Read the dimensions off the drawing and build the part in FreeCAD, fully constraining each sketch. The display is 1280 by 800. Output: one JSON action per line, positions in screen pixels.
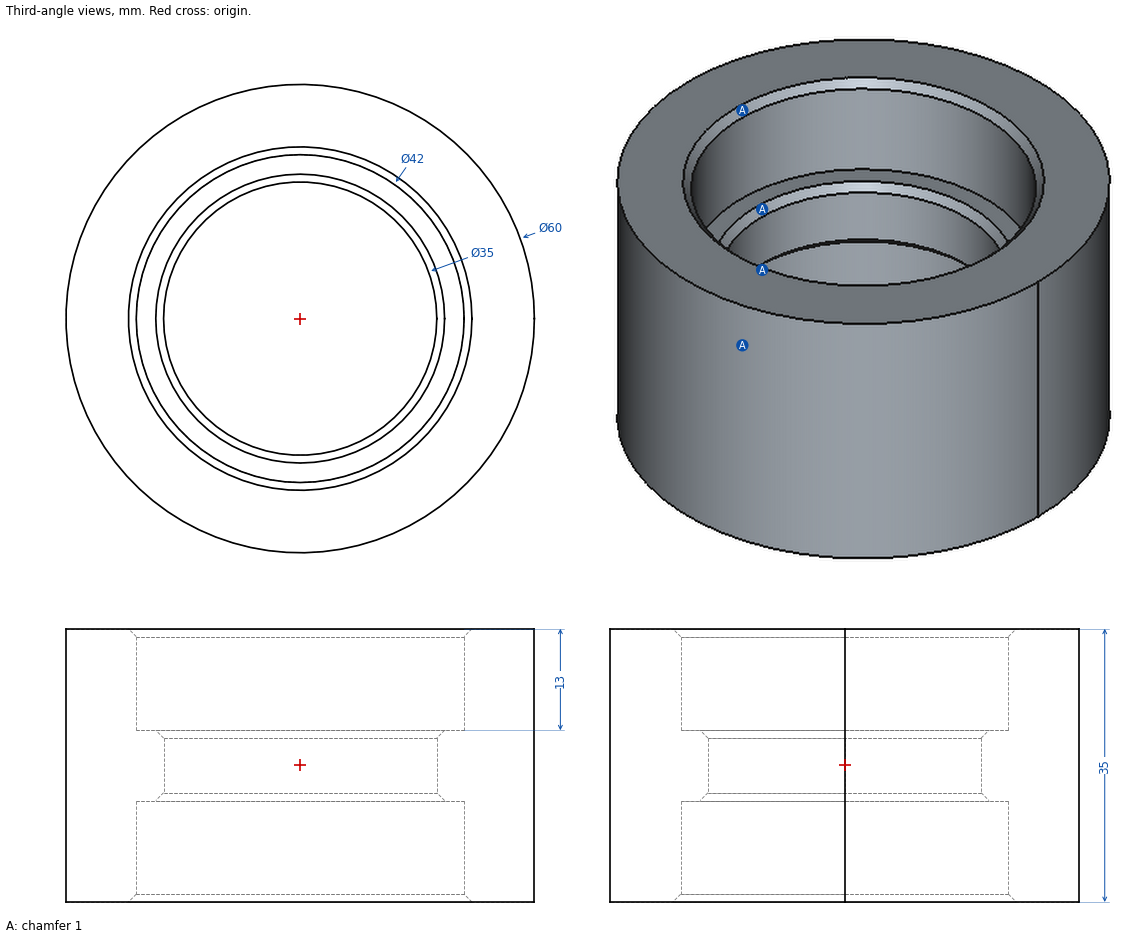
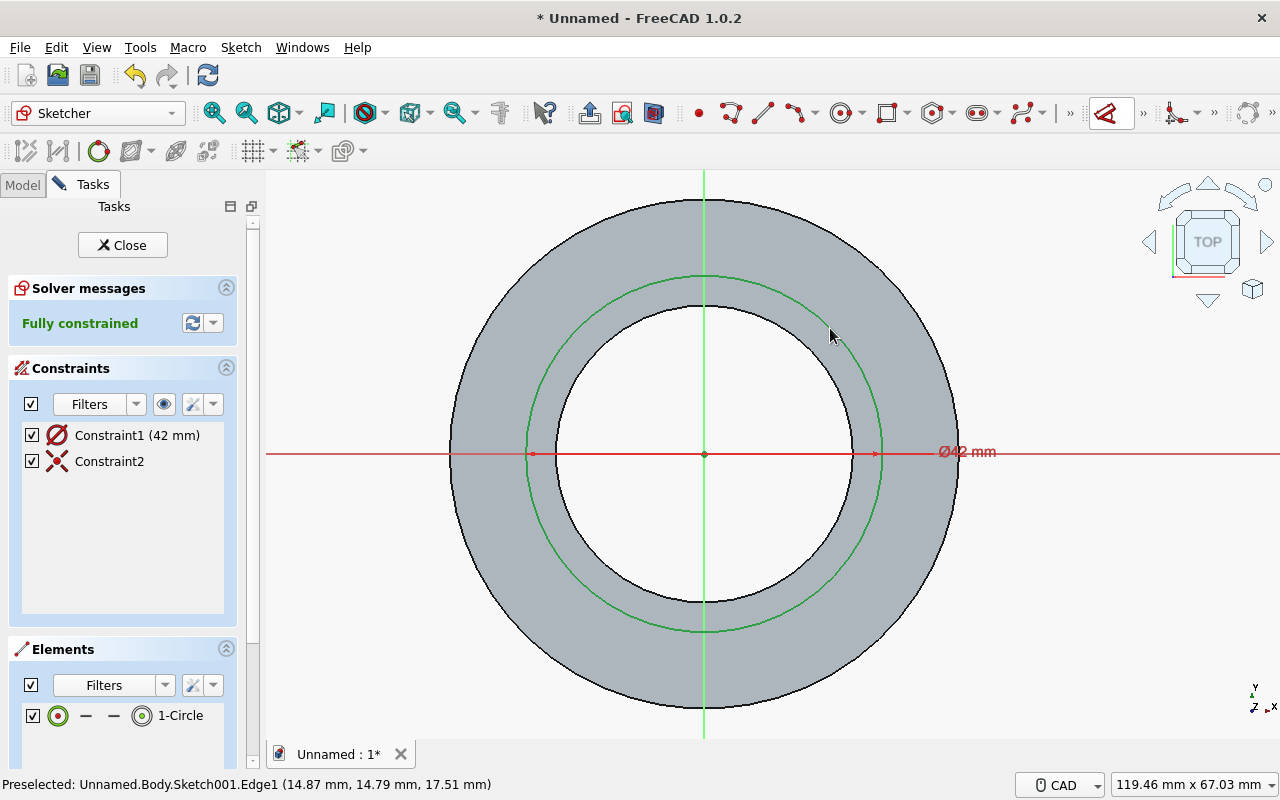
{"action": "left_click", "coordinate": [123, 245]}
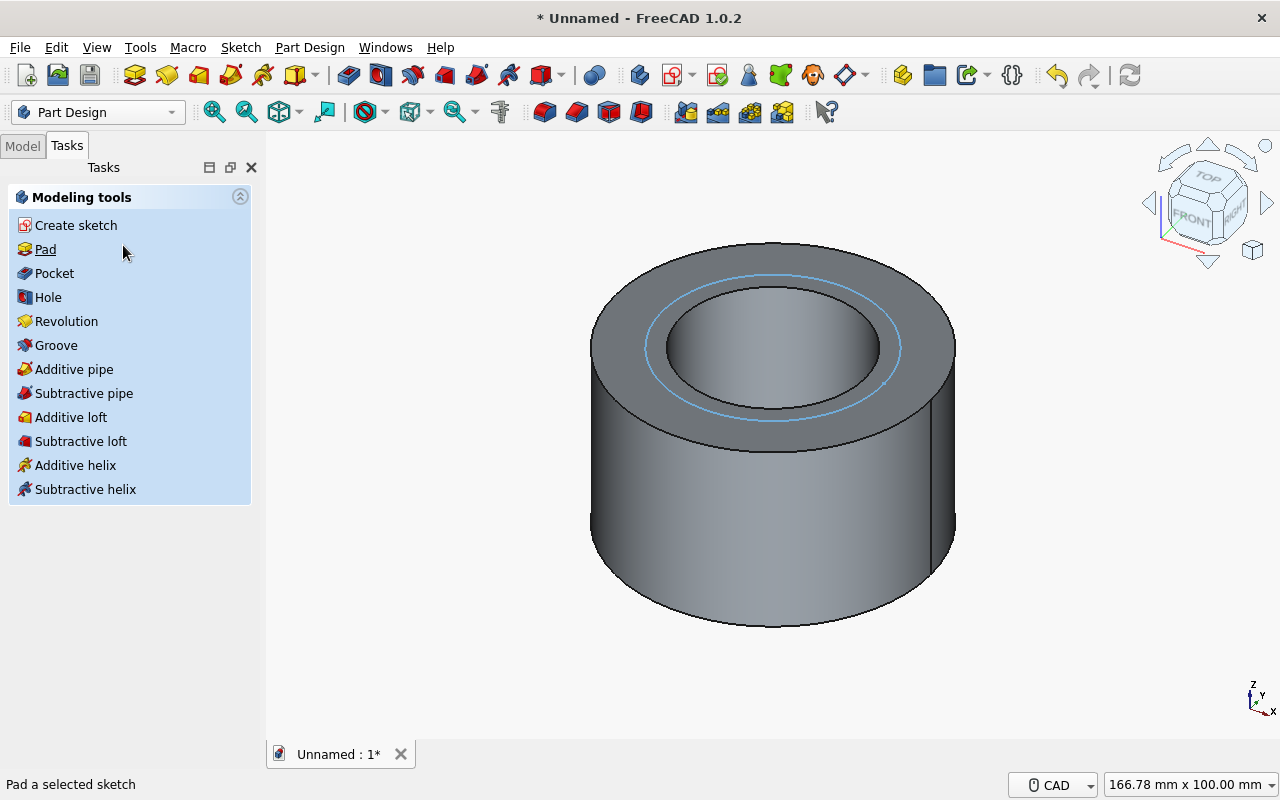
{"action": "left_click", "coordinate": [350, 76]}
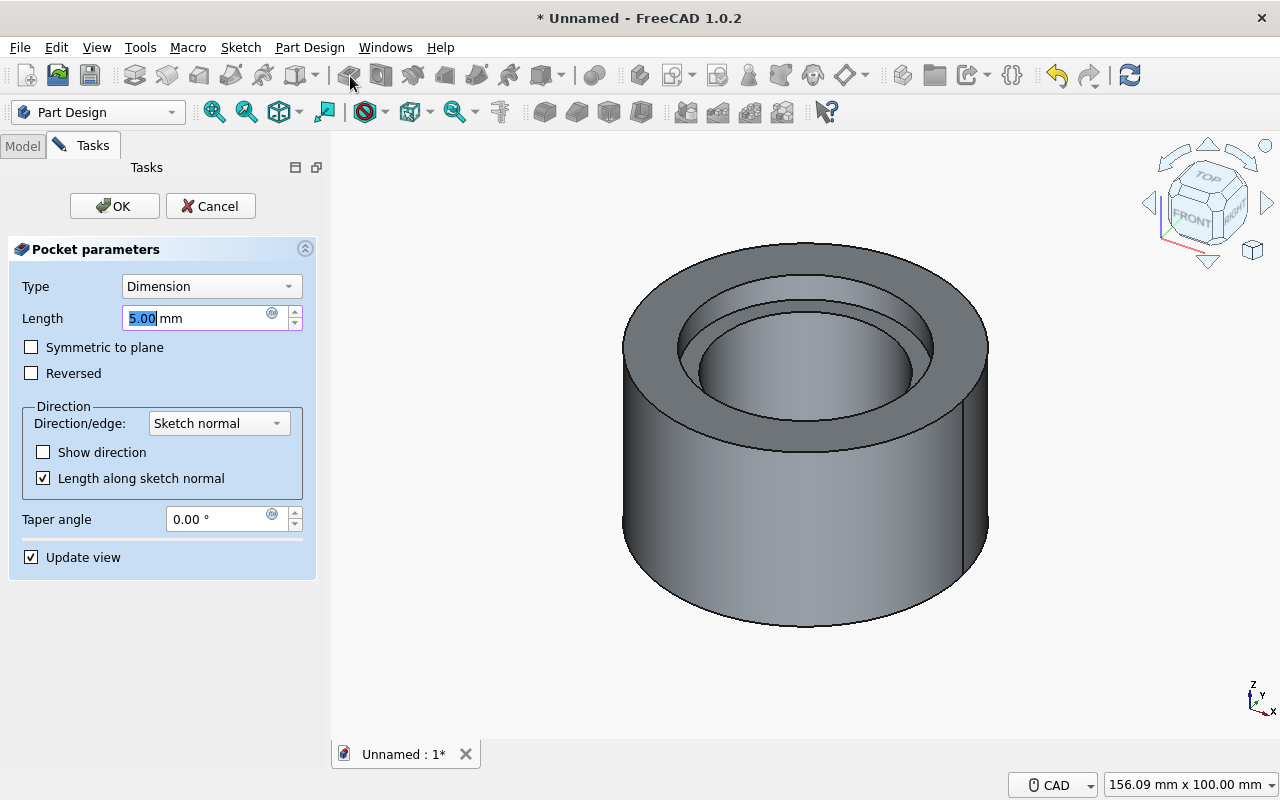
{"action": "type", "text": "13"}
{"action": "key", "text": "Tab"}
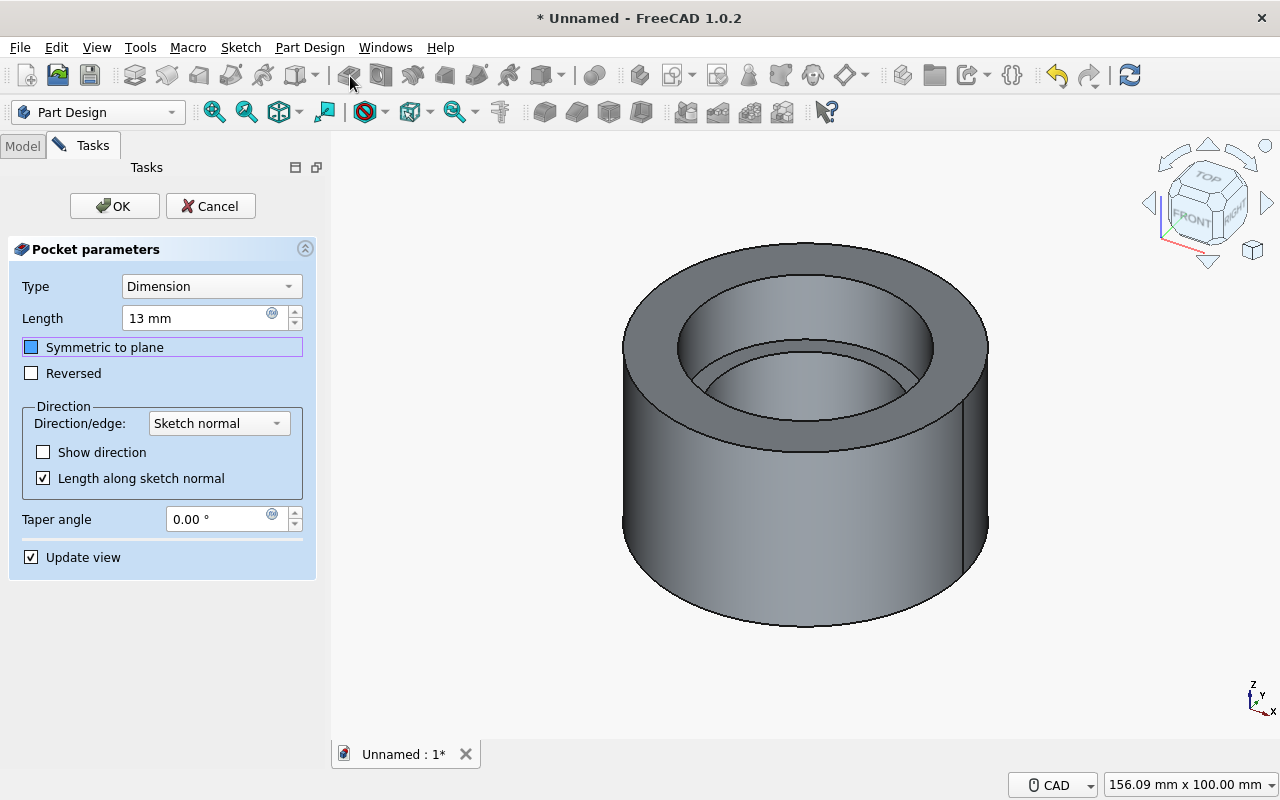
{"action": "left_click", "coordinate": [115, 206]}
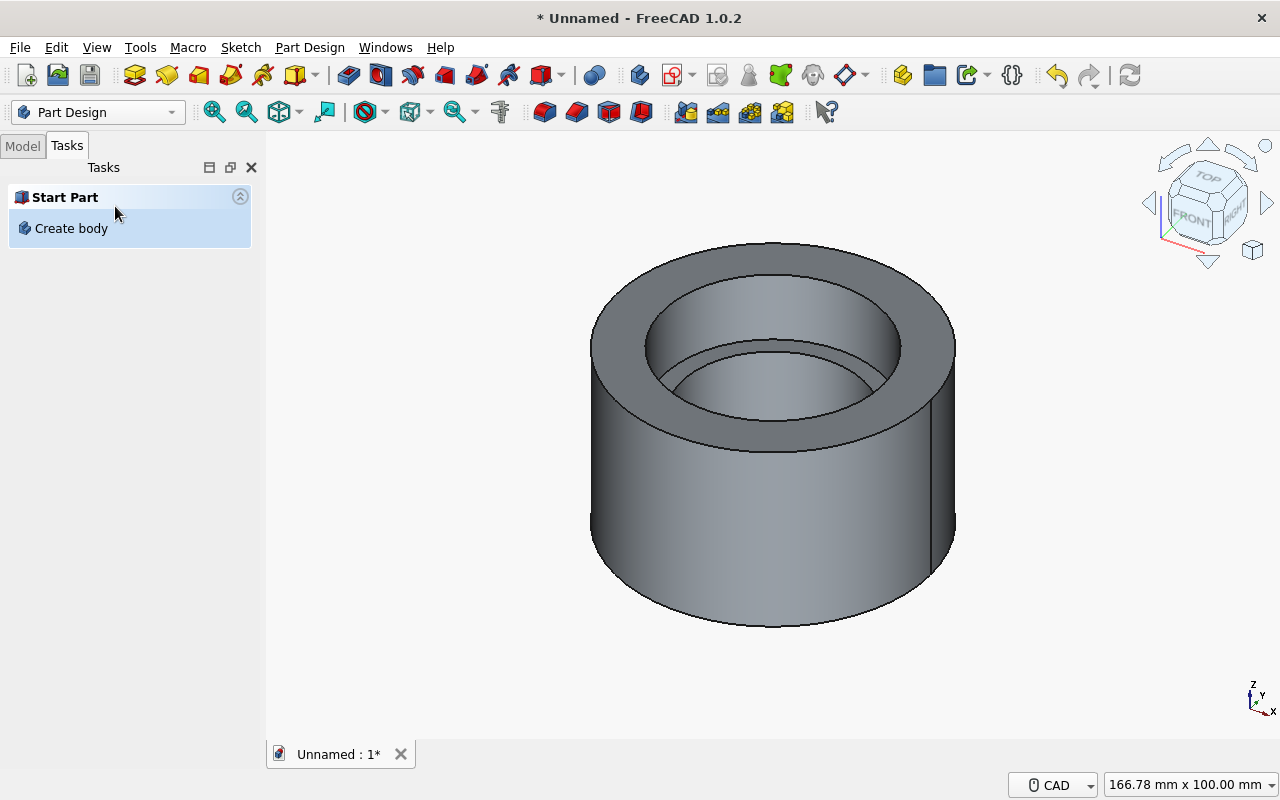
{"action": "left_click", "coordinate": [23, 145]}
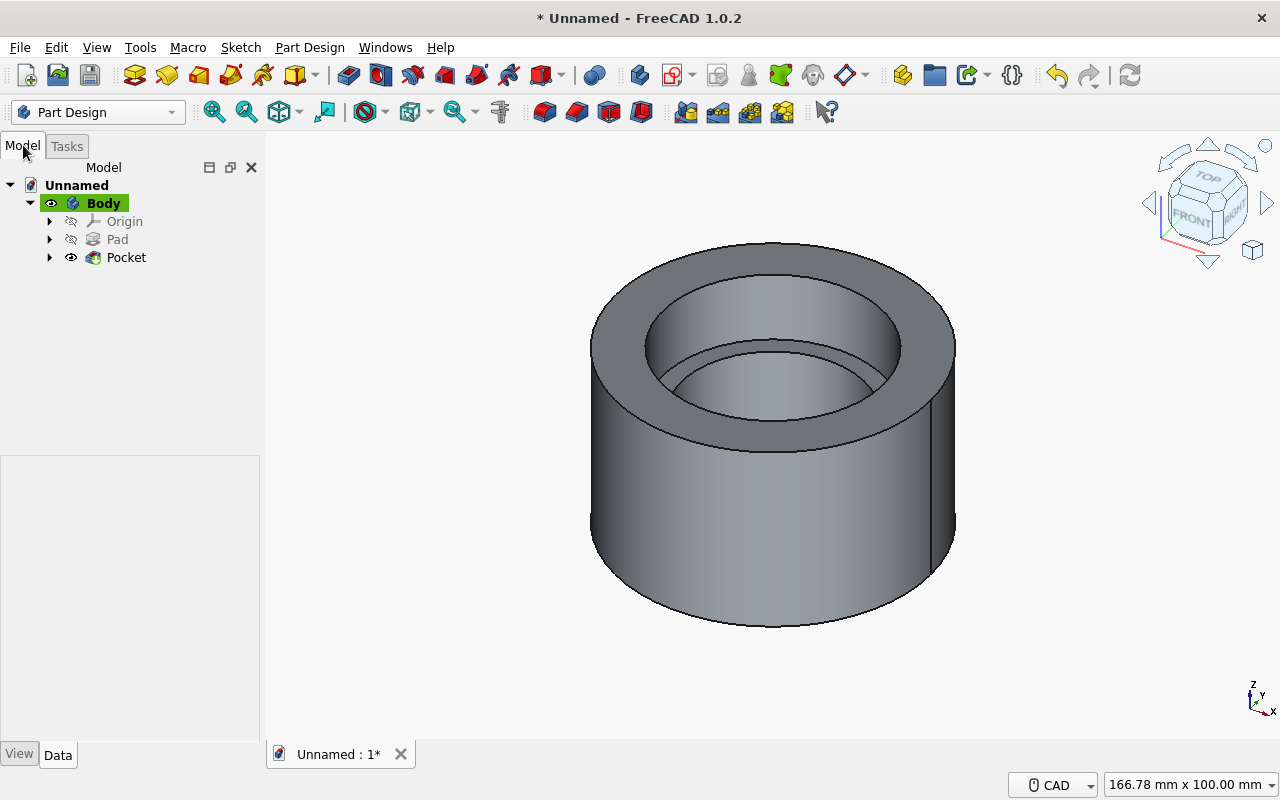
{"action": "left_click", "coordinate": [116, 257]}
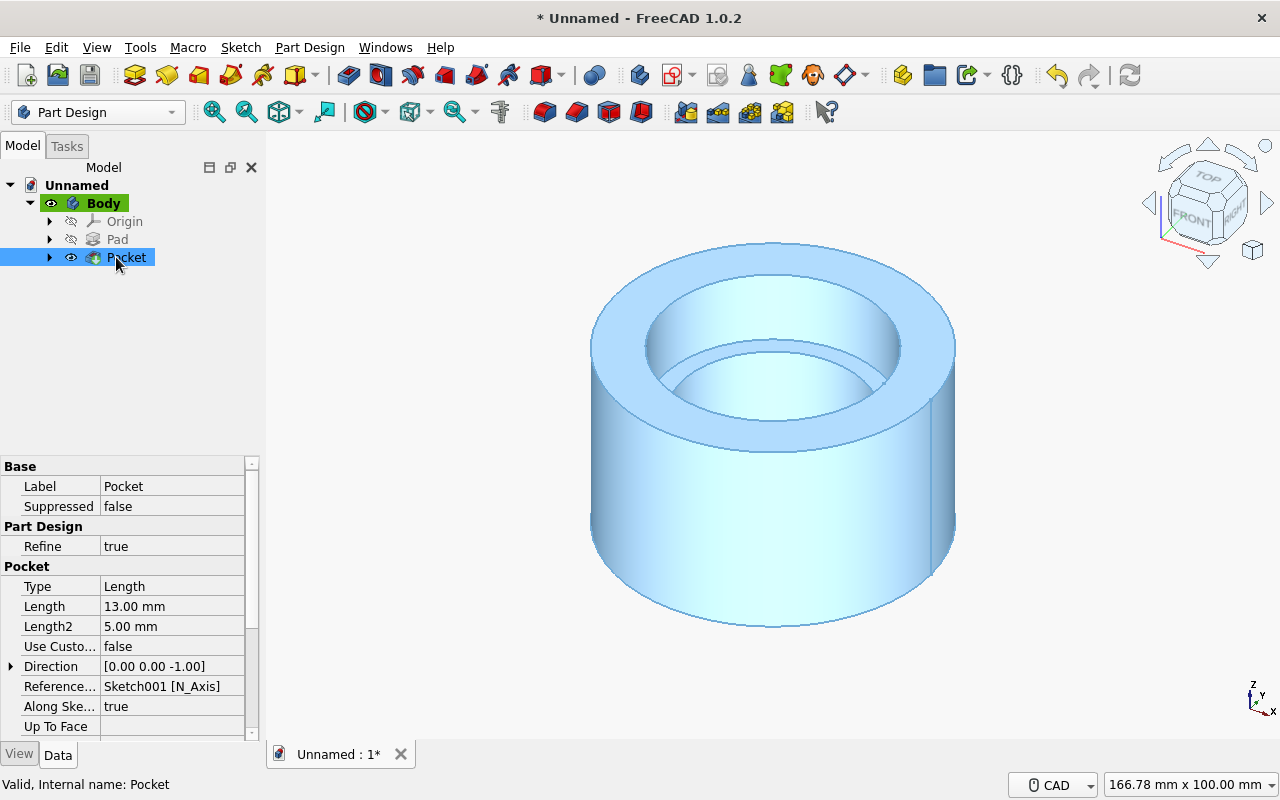
{"action": "left_click", "coordinate": [686, 112]}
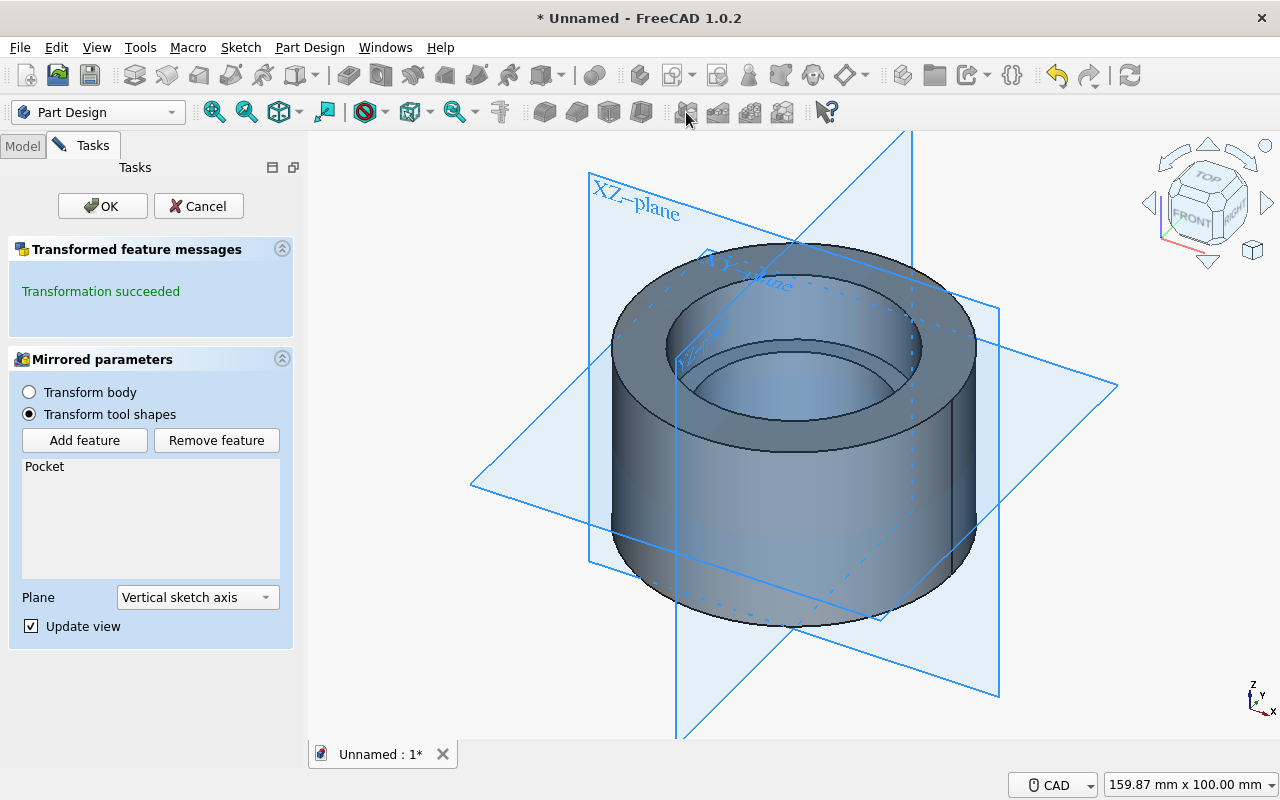
{"action": "left_click", "coordinate": [198, 598]}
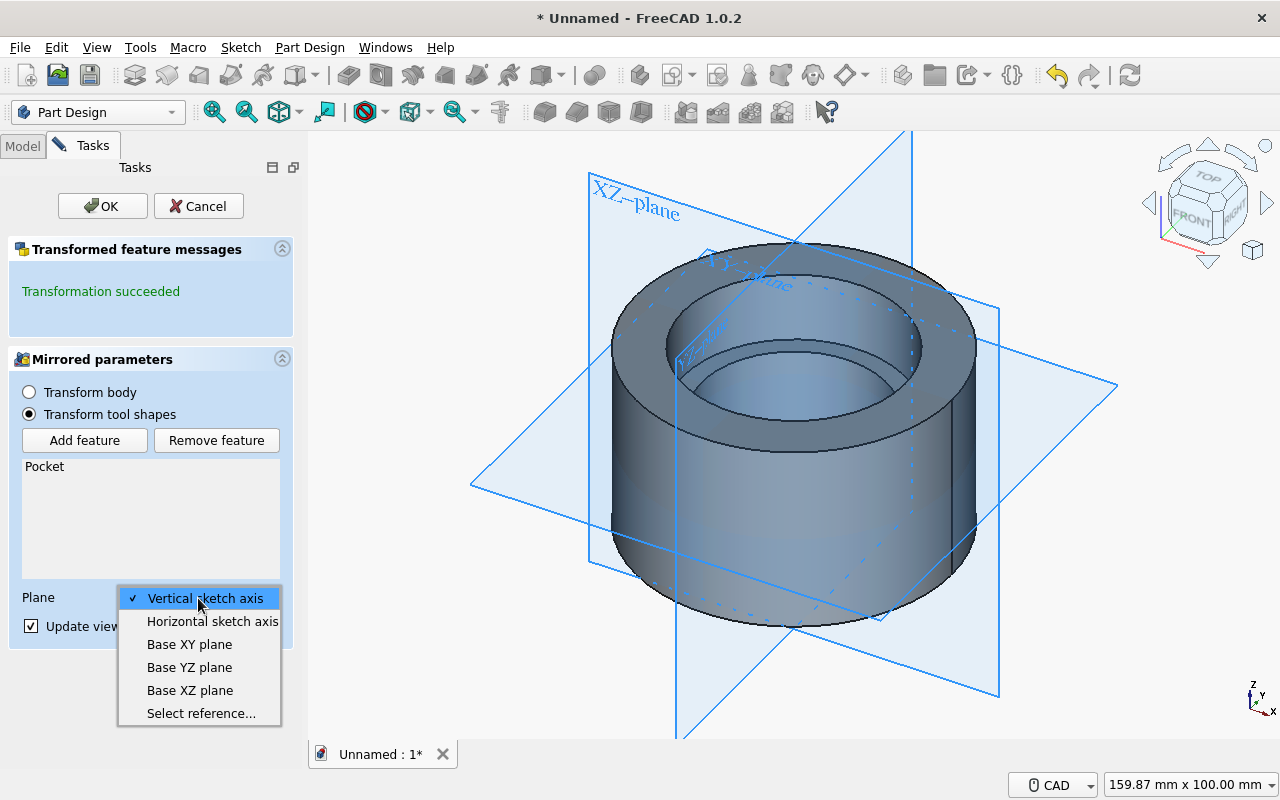
{"action": "left_click", "coordinate": [198, 644]}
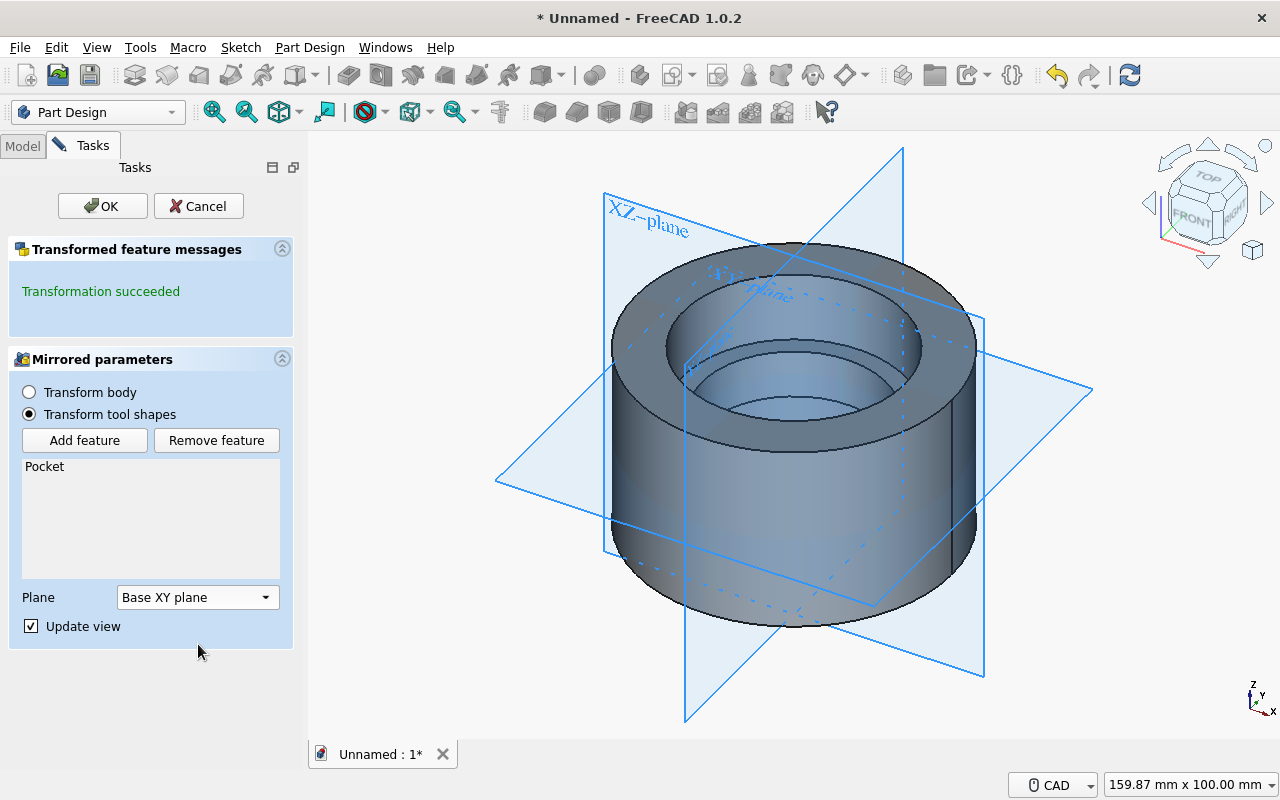
{"action": "left_click", "coordinate": [103, 206]}